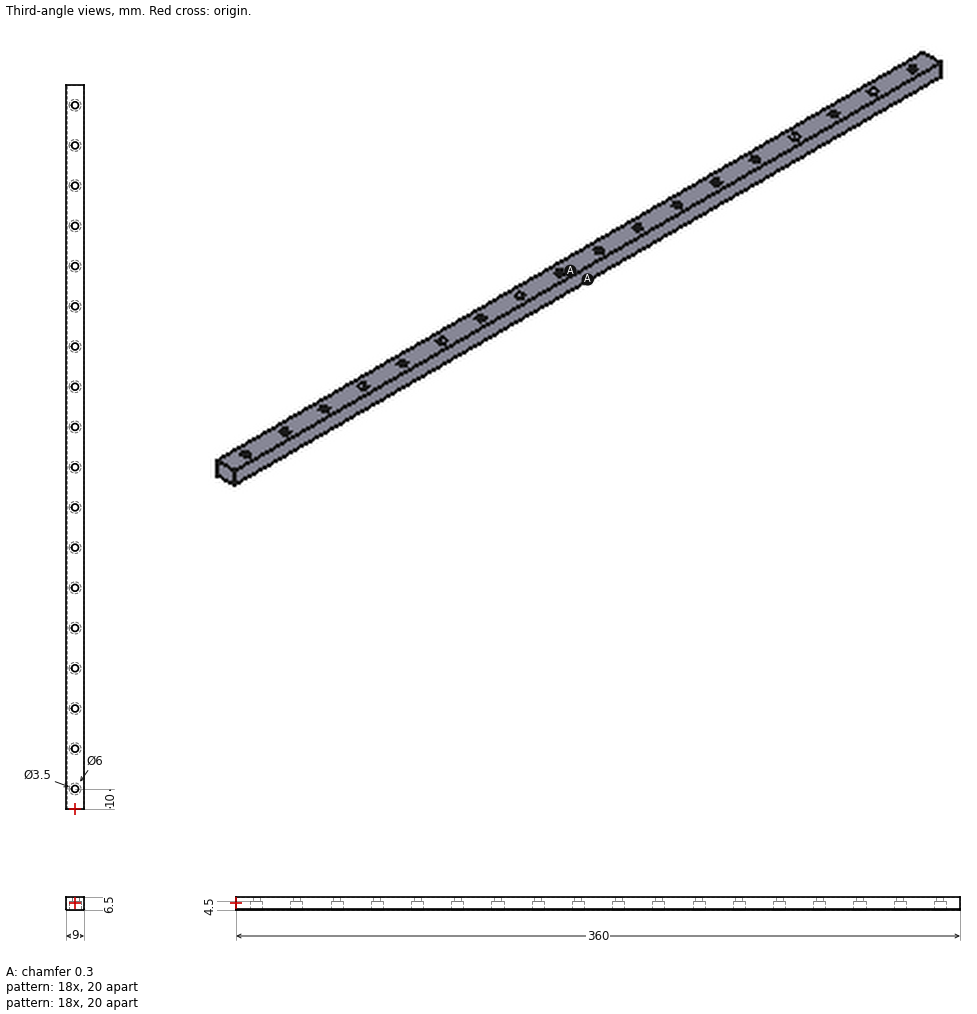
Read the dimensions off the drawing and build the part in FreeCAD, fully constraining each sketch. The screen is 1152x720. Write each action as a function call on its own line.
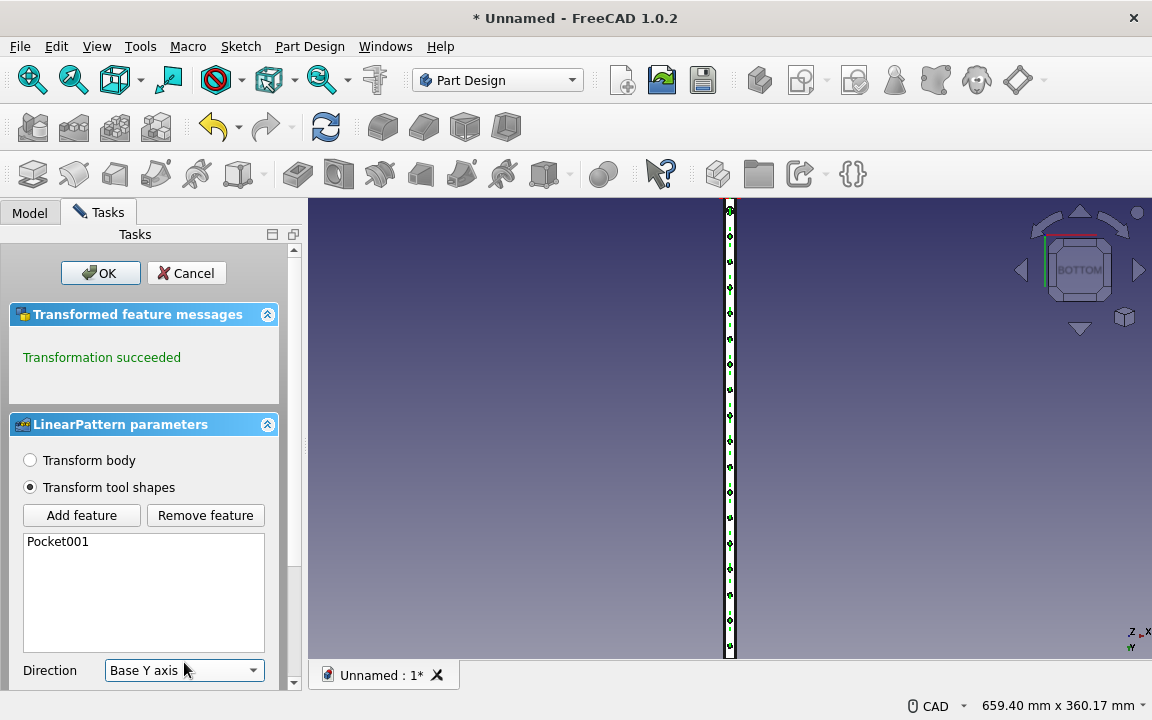
scroll(294, 467, down, 2)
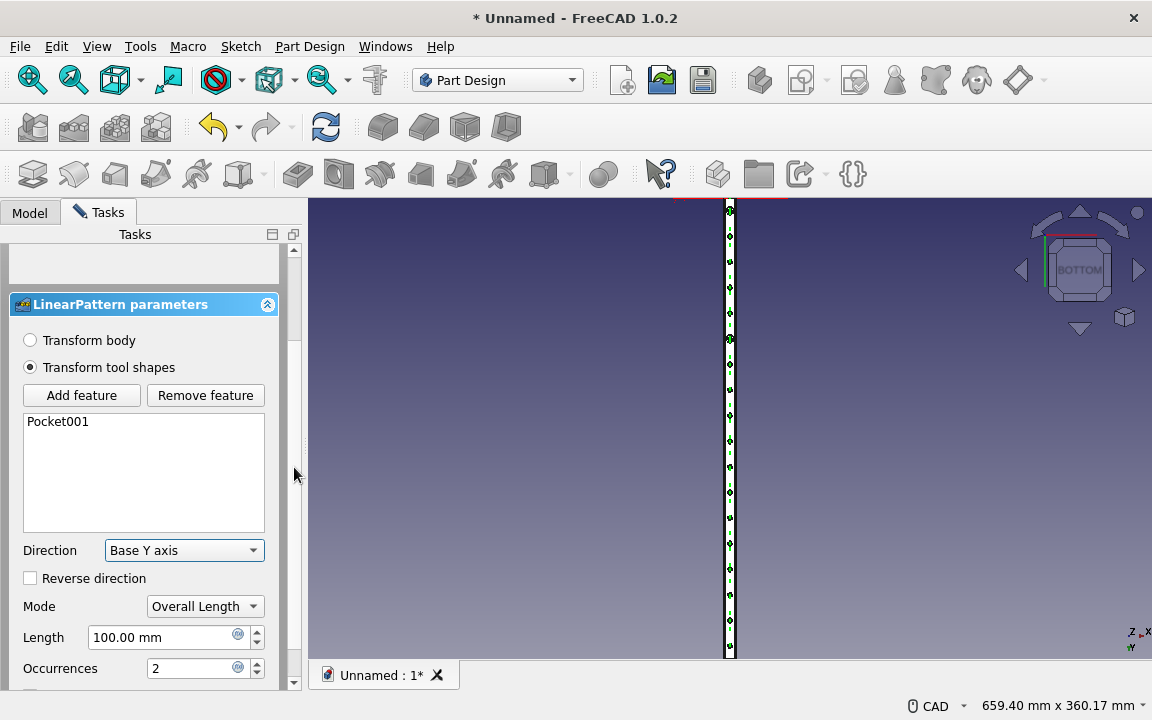
click(206, 606)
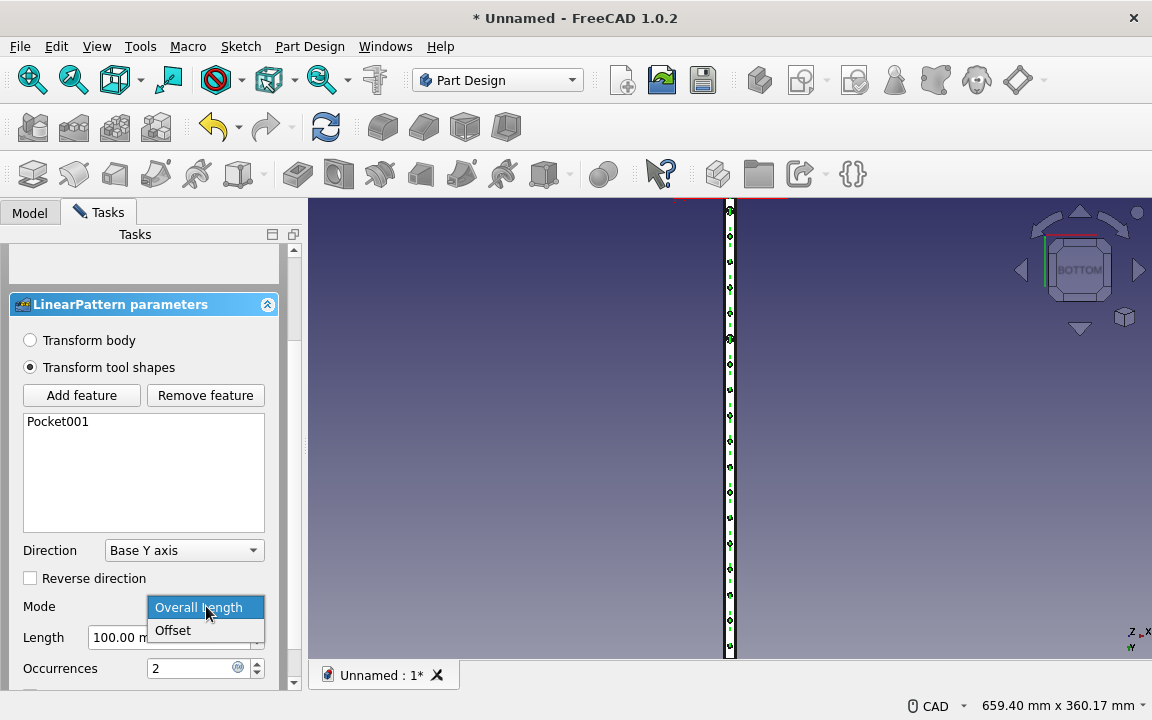
click(204, 630)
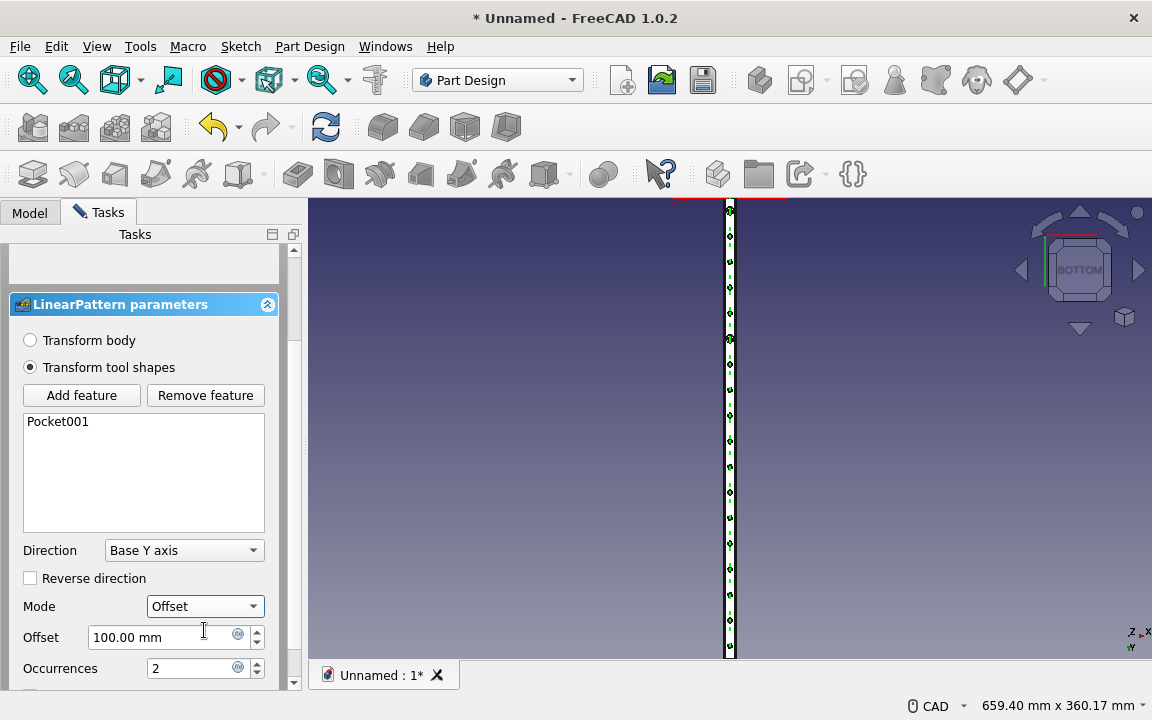
triple_click(170, 638)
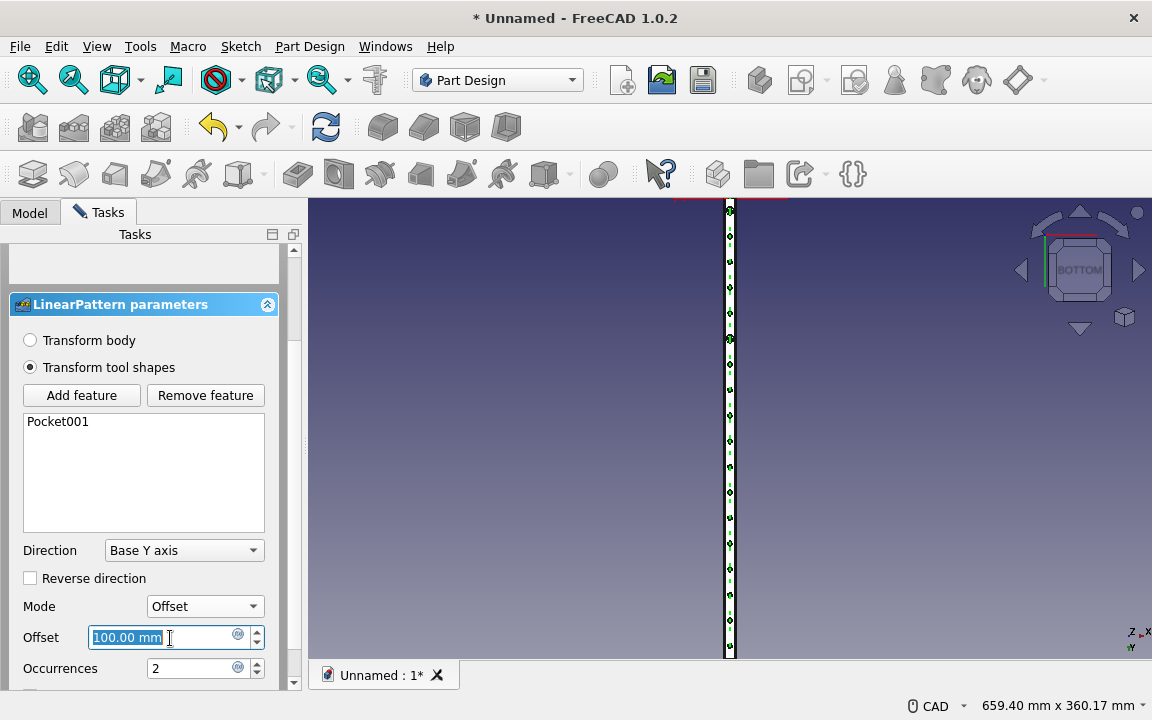
text(20)
key(Tab)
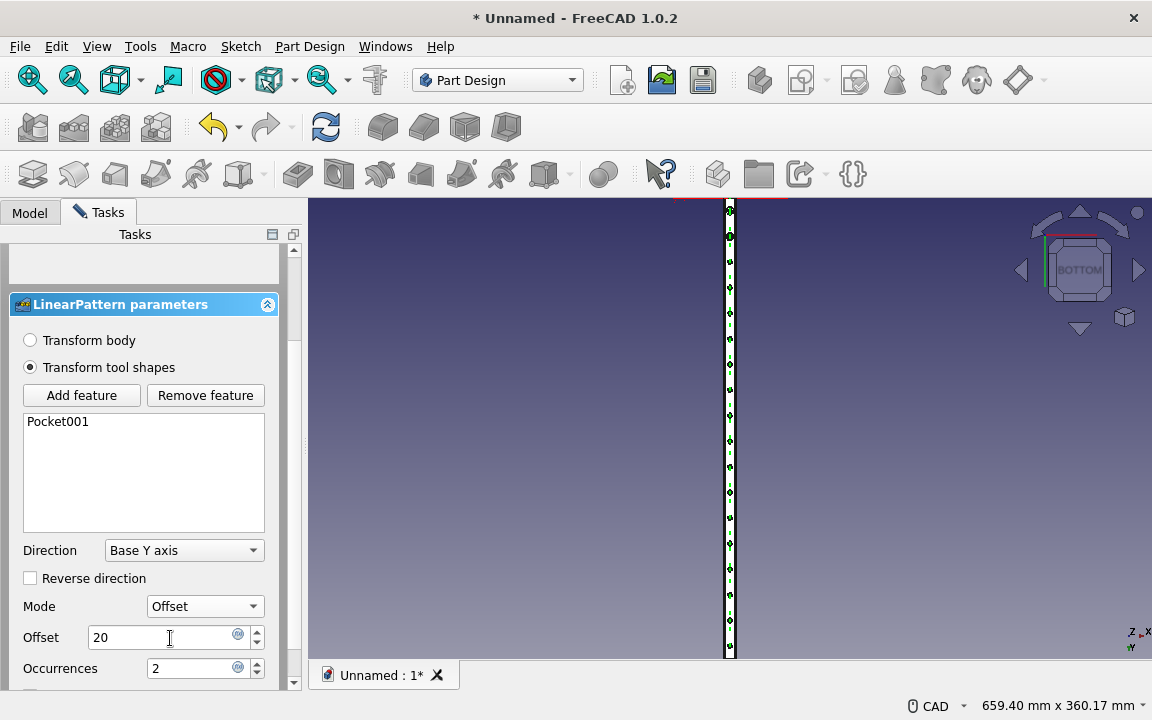
triple_click(199, 668)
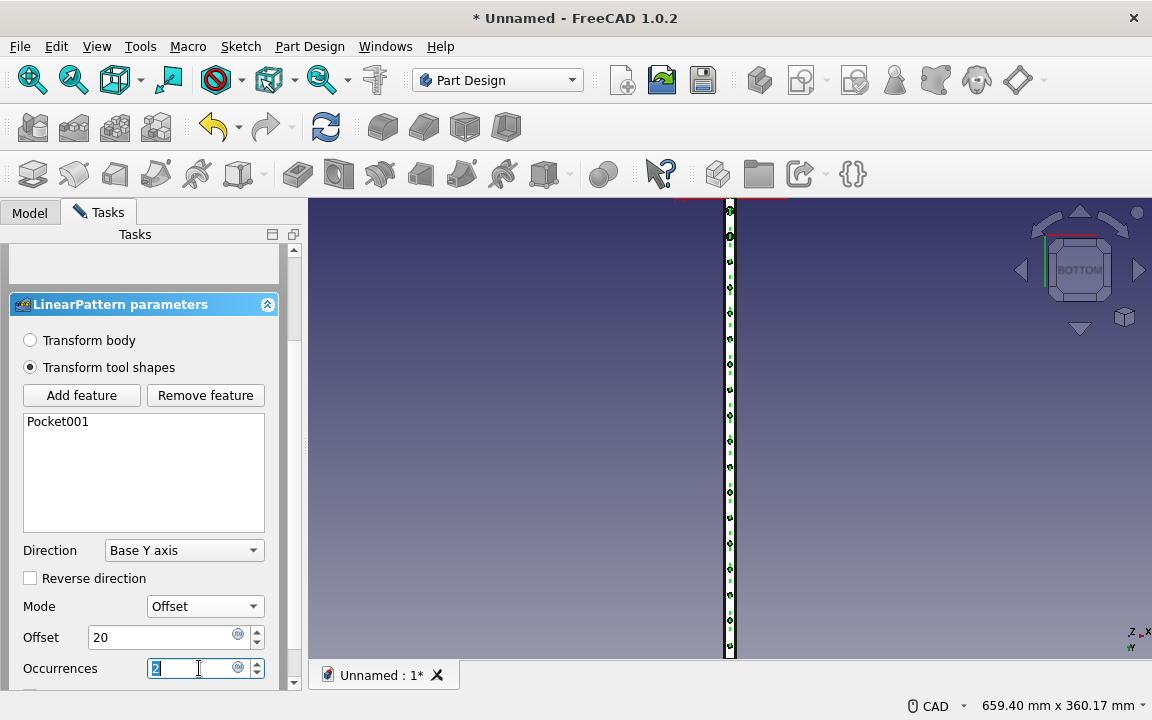
text(18)
key(Tab)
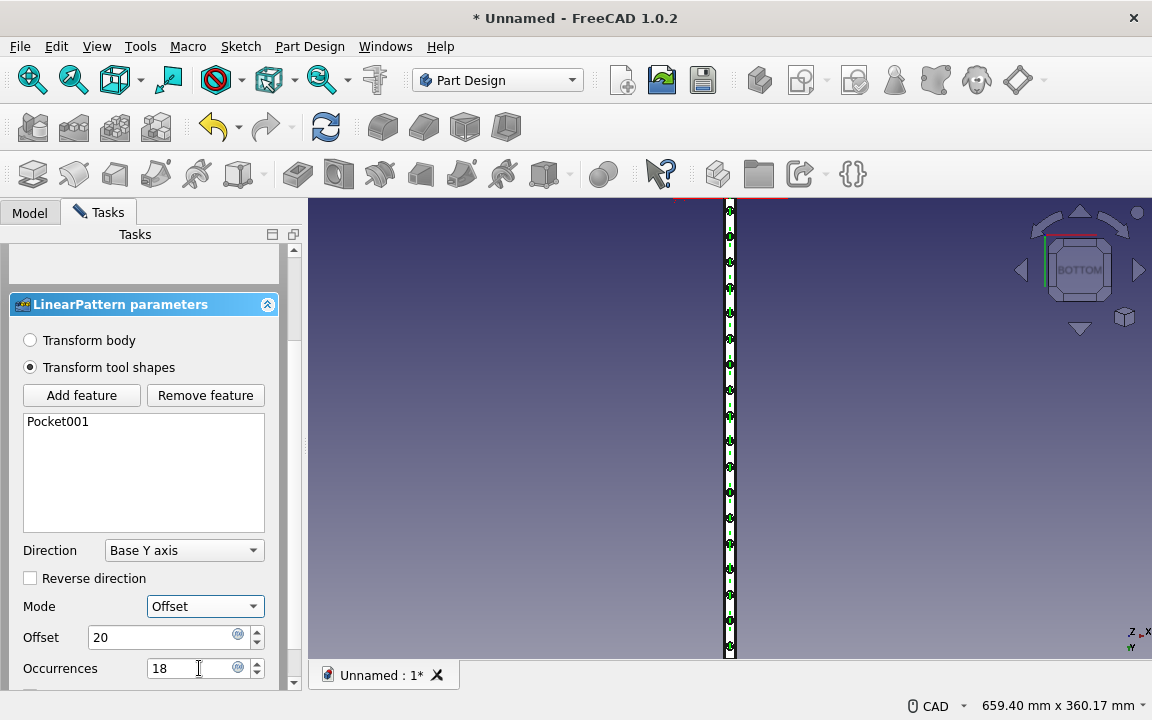
scroll(294, 467, up, 3)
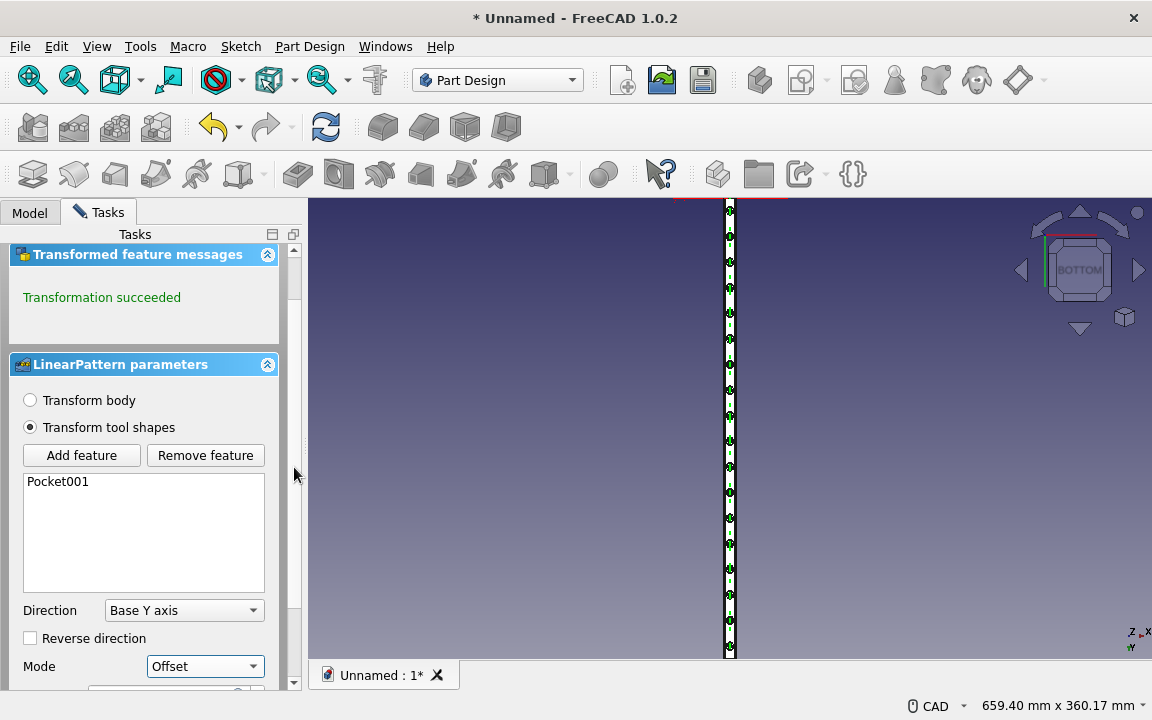
click(101, 273)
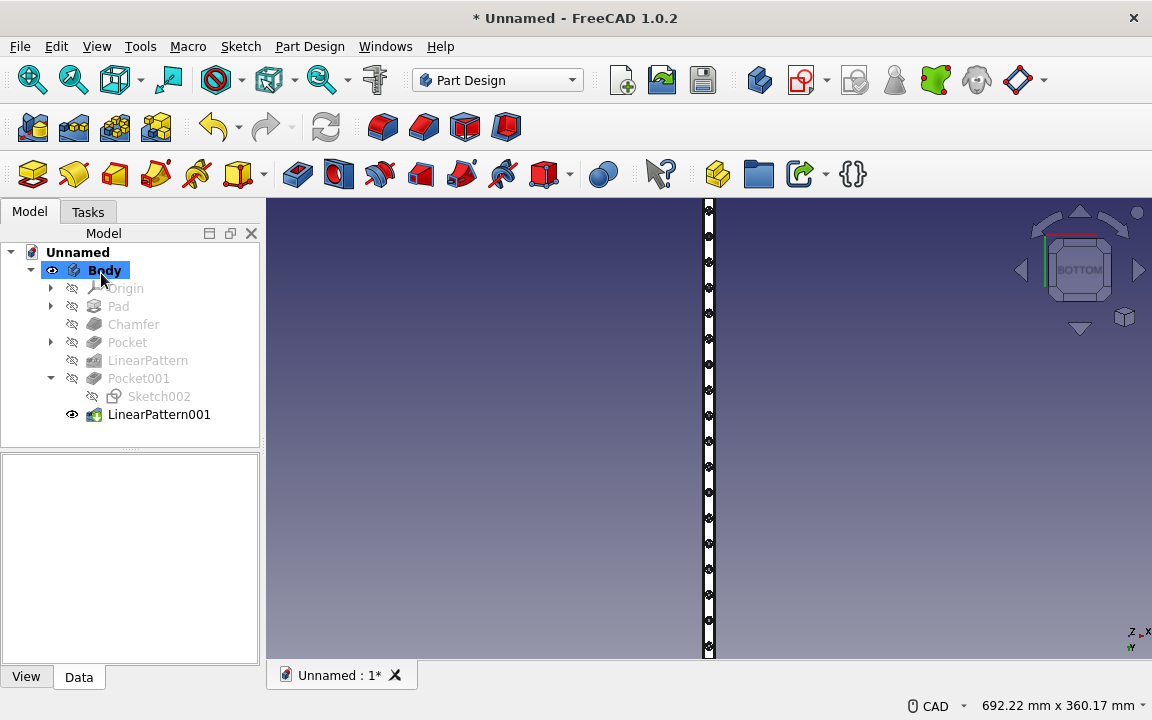
key(0)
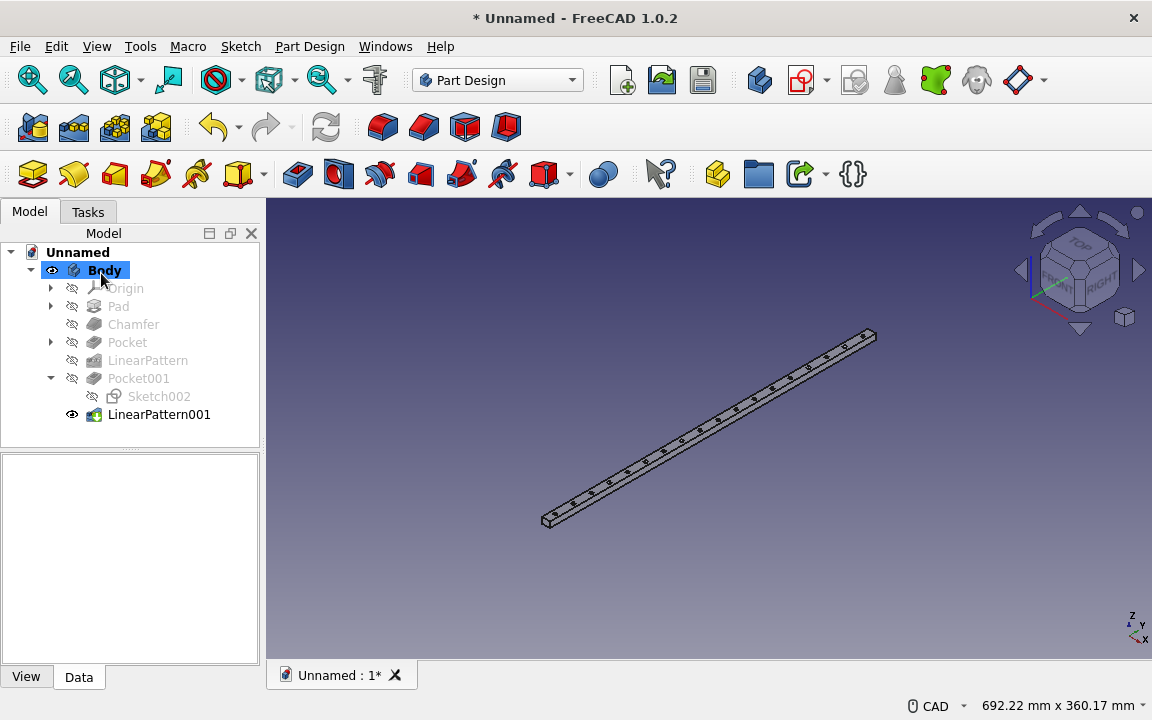
key(v)
key(f)